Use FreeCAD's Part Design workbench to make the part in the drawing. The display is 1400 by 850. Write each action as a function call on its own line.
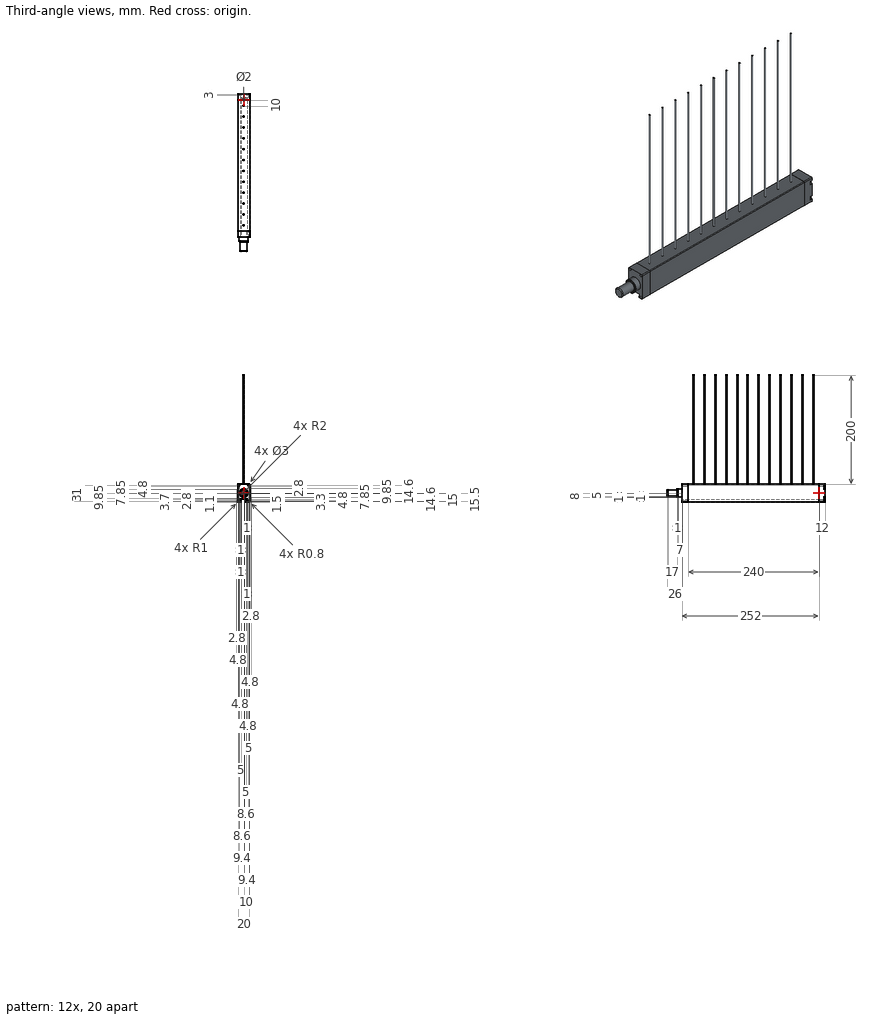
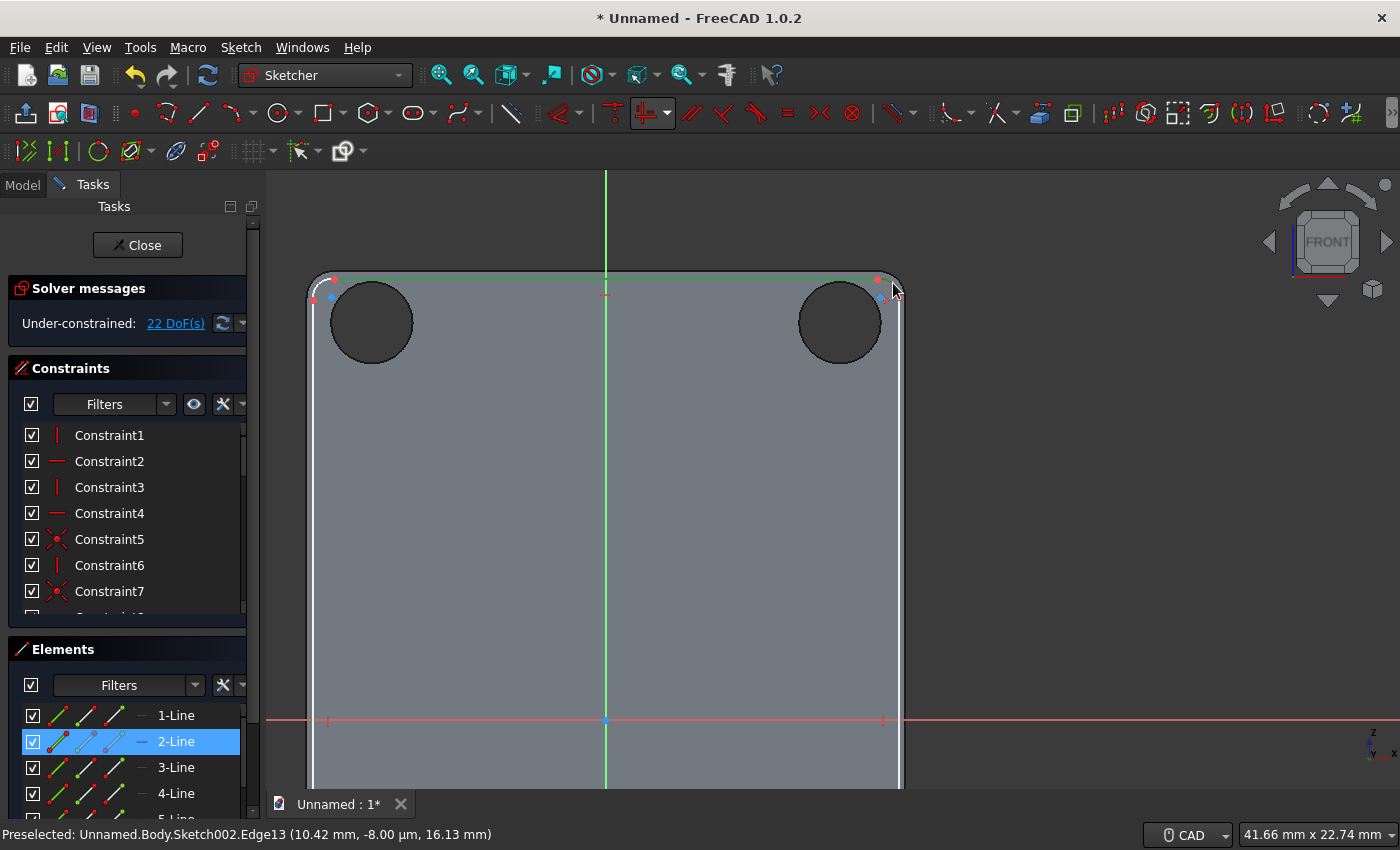
click(756, 114)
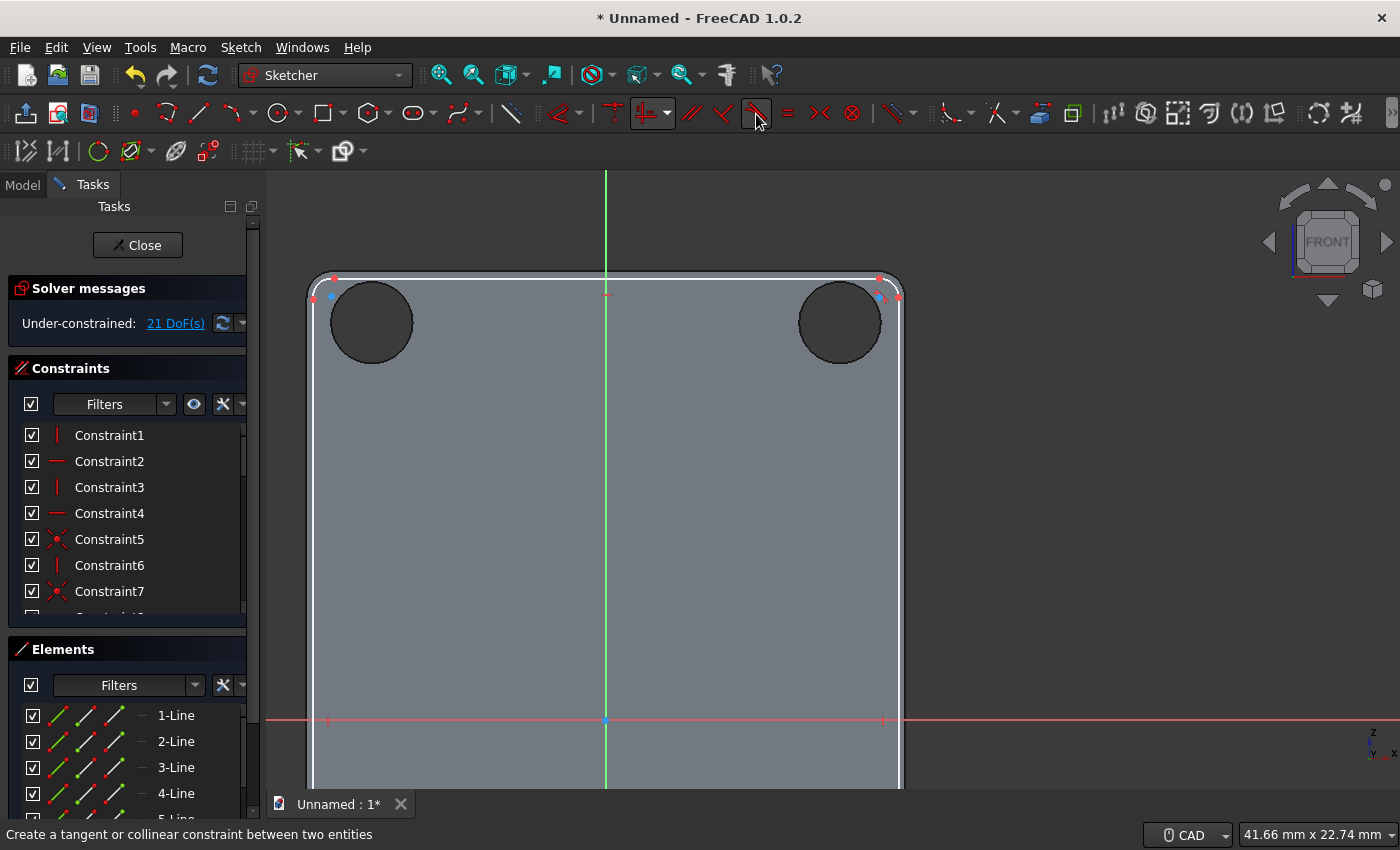
click(716, 279)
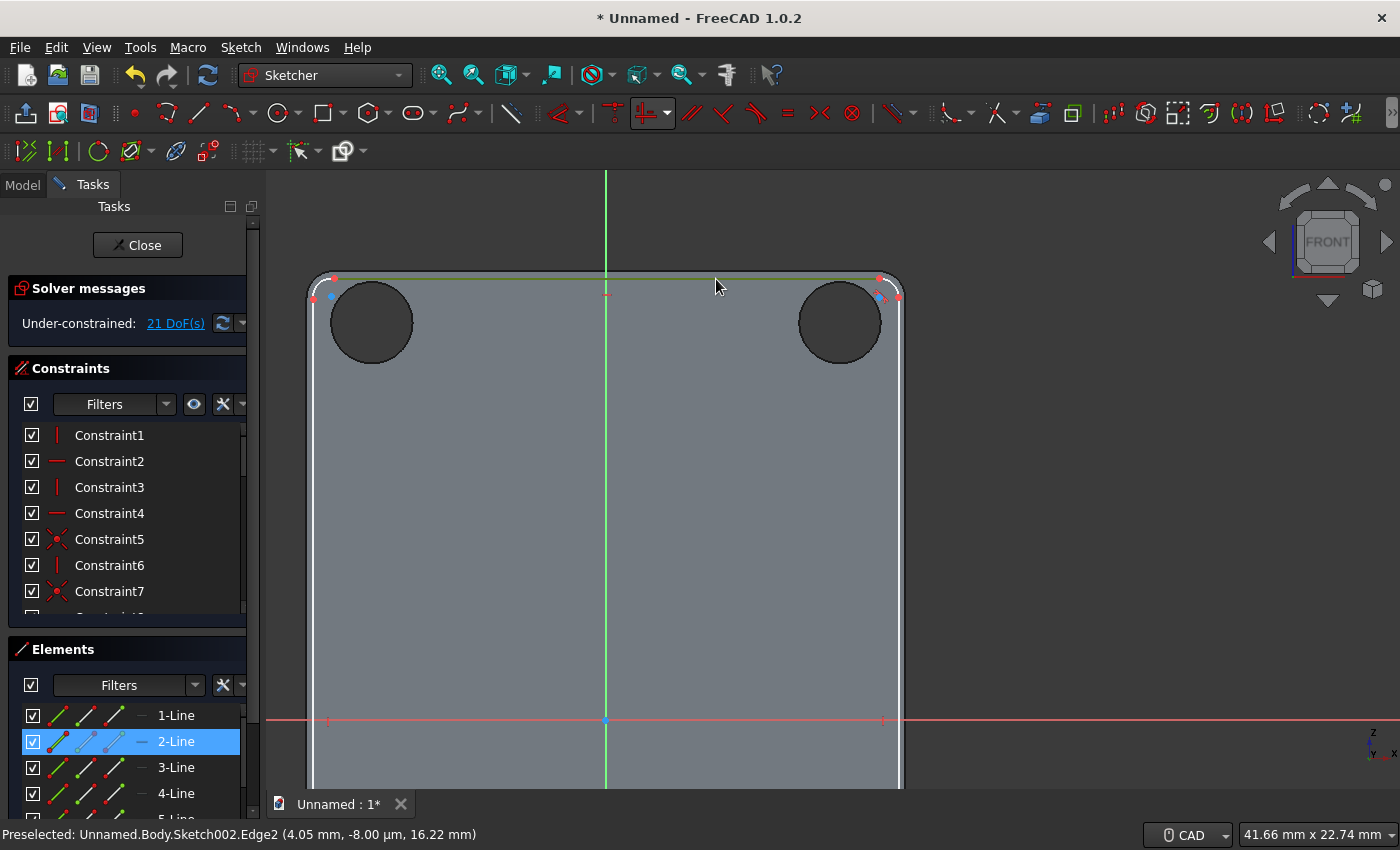
scroll(324, 280, up, 2)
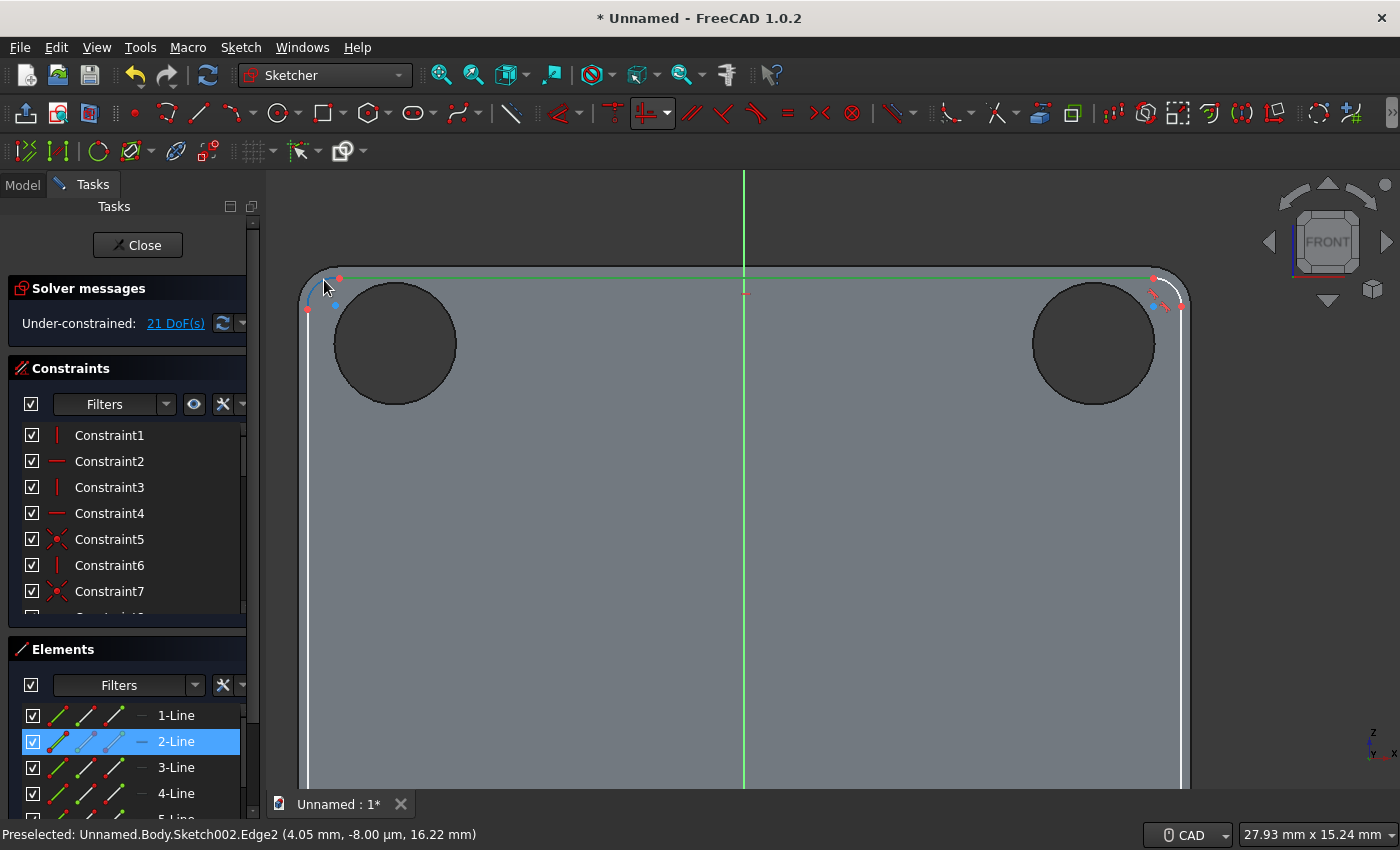
click(324, 280)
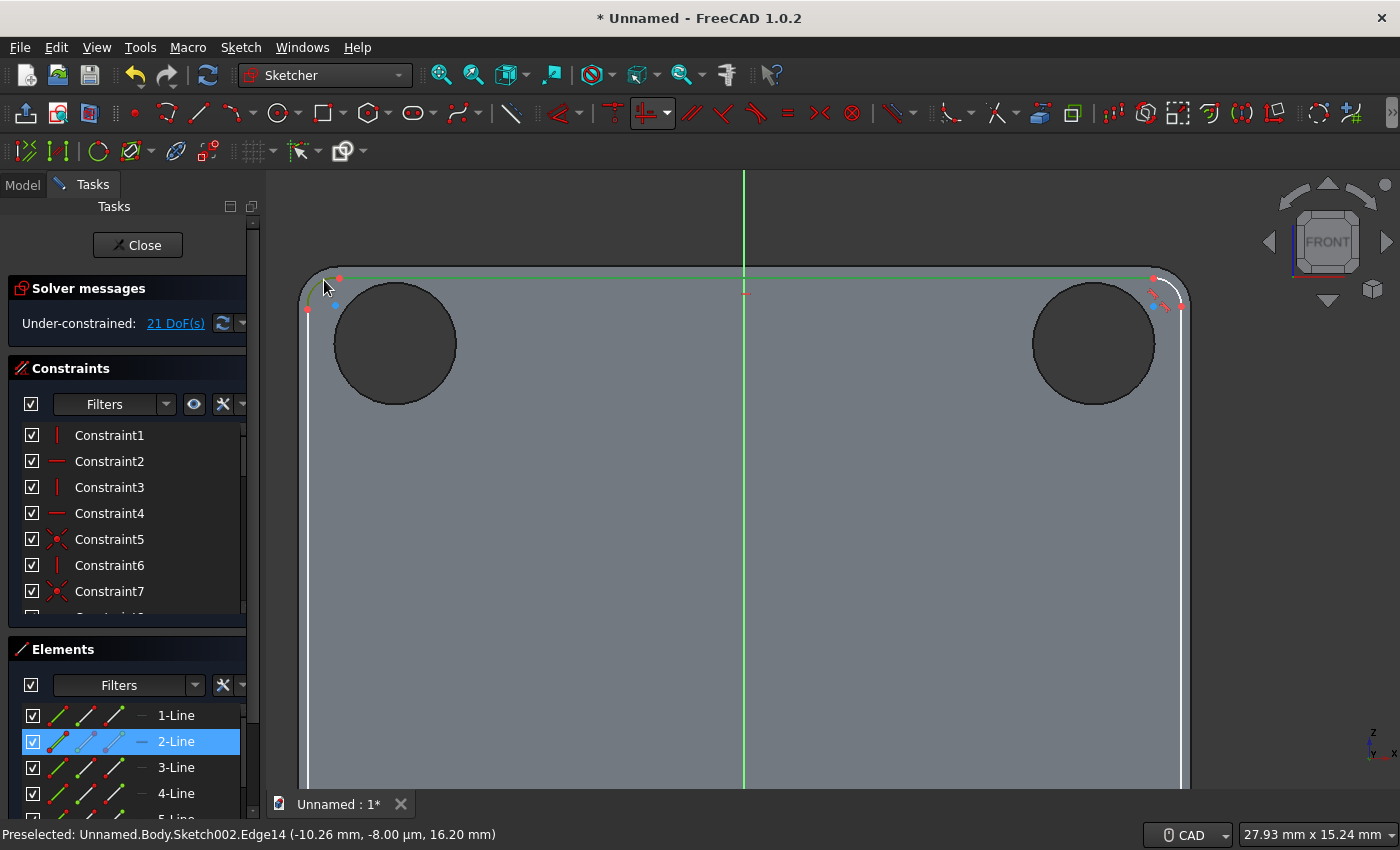
click(756, 114)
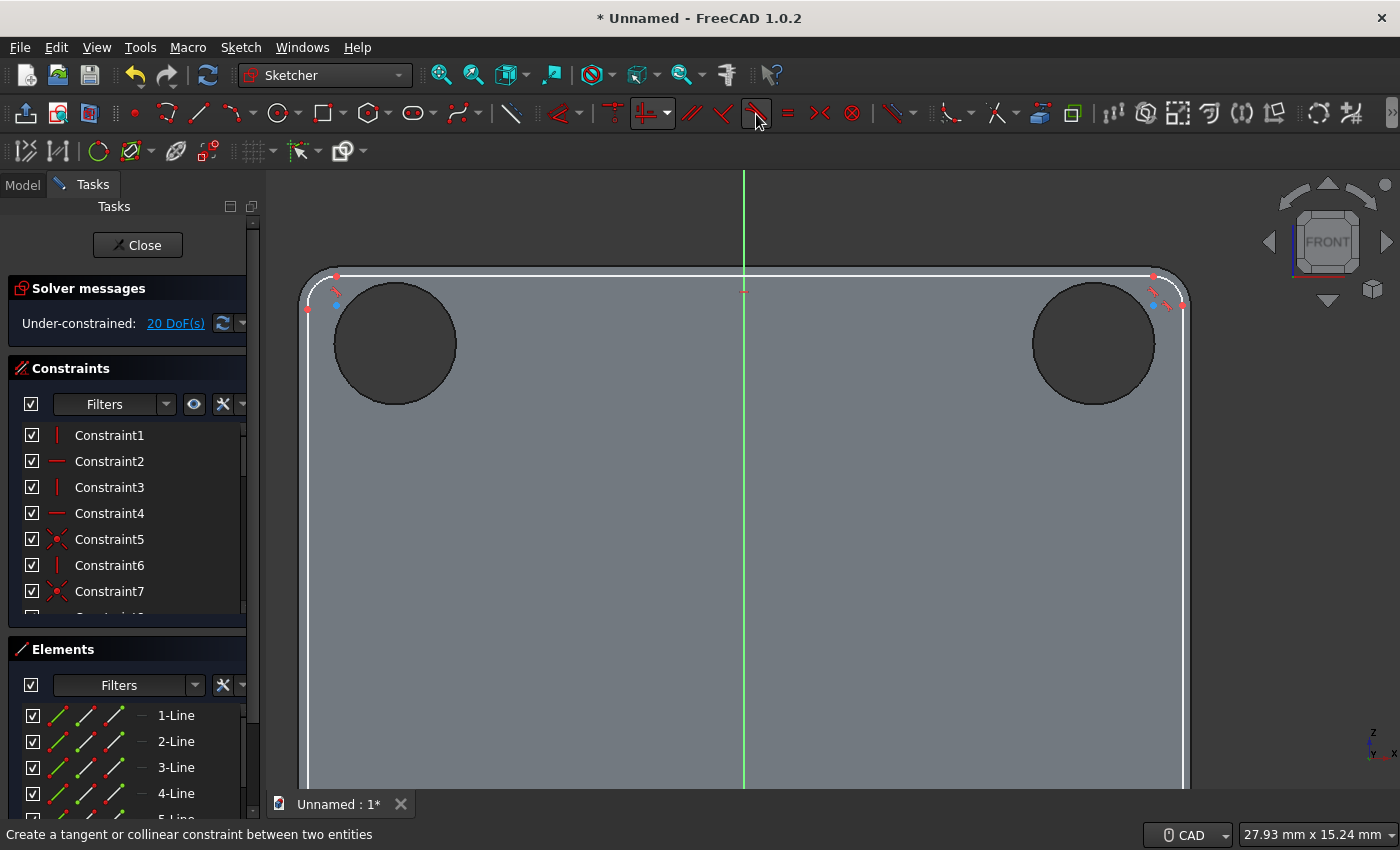
click(308, 687)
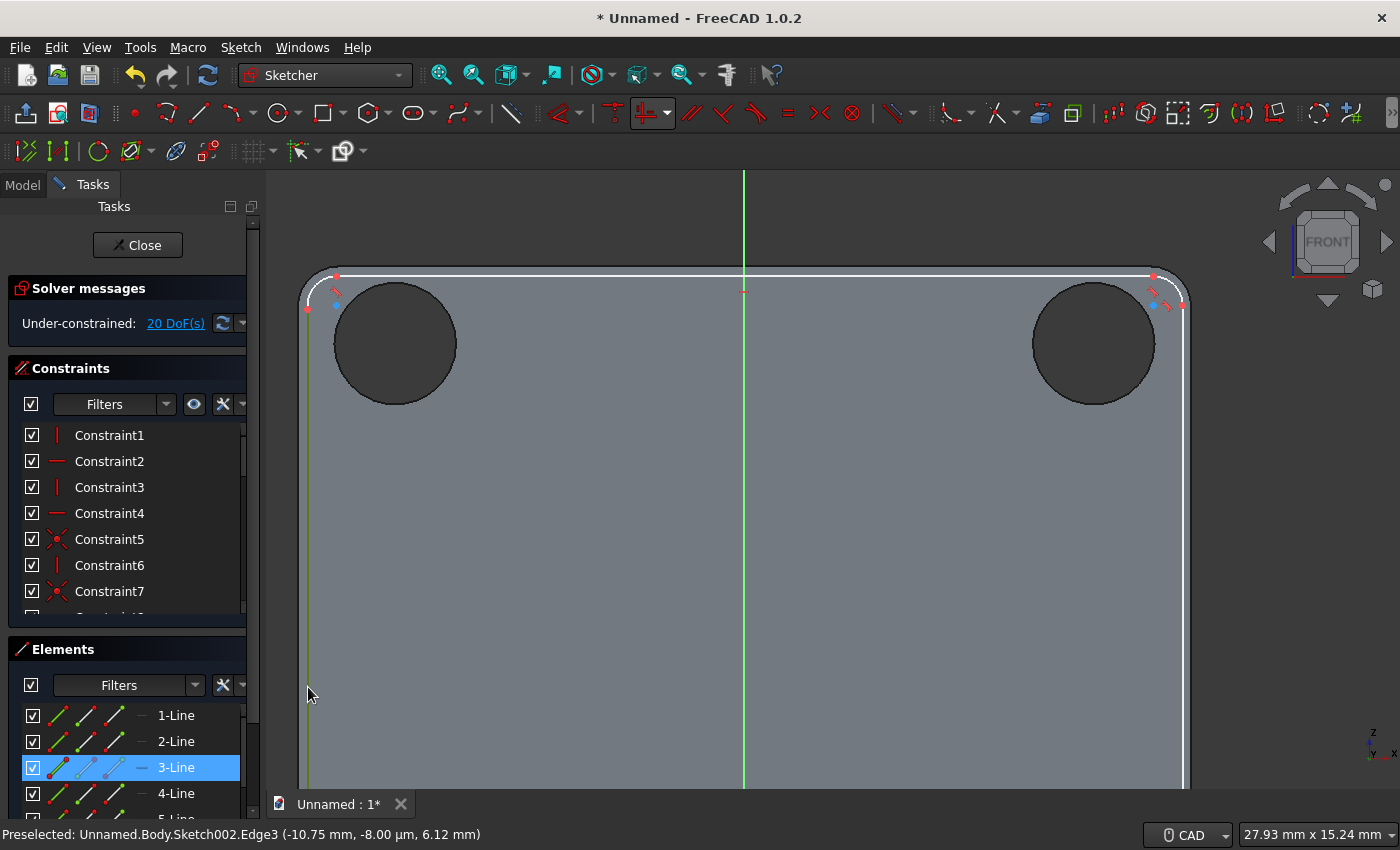
click(322, 280)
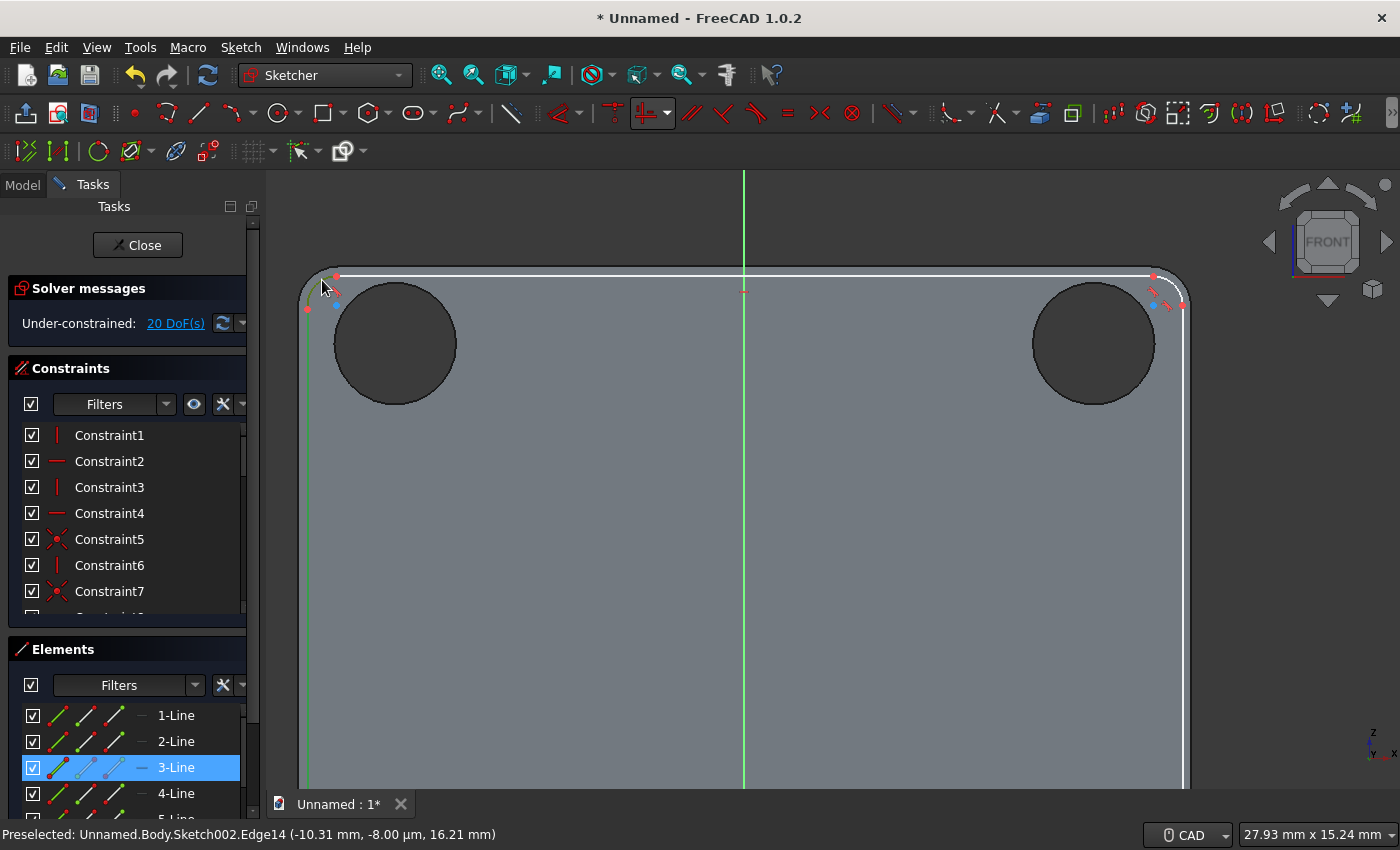
click(756, 114)